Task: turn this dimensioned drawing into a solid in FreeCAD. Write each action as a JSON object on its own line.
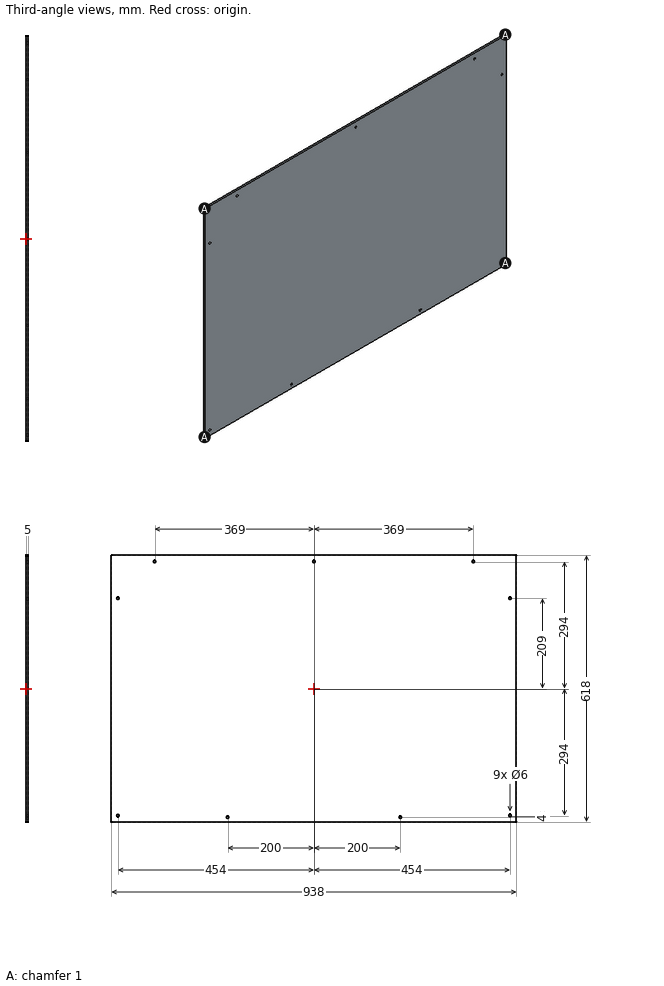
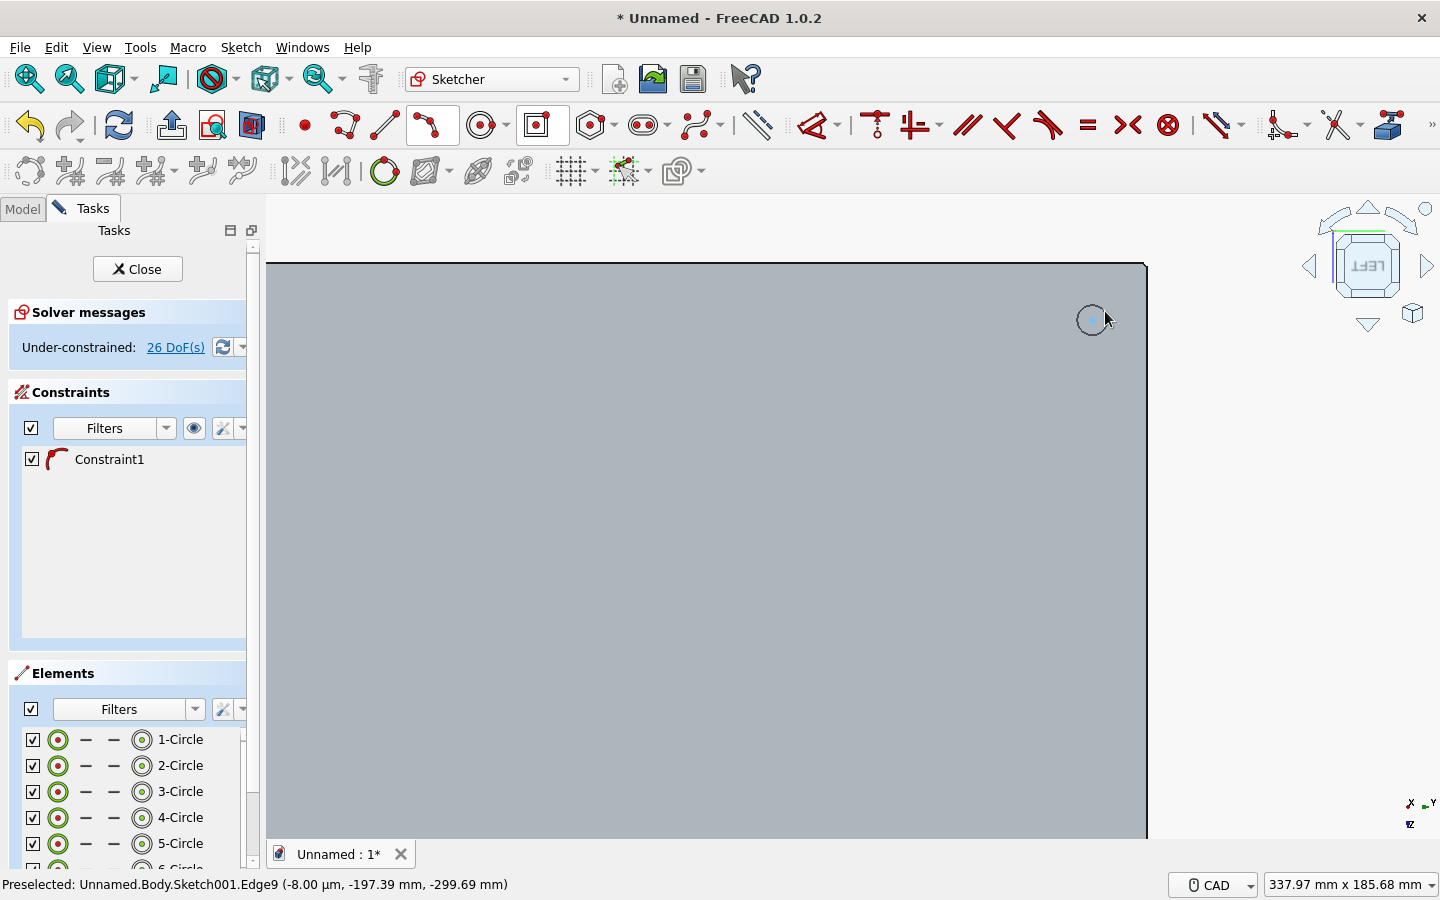
{"action": "left_click", "coordinate": [1103, 310]}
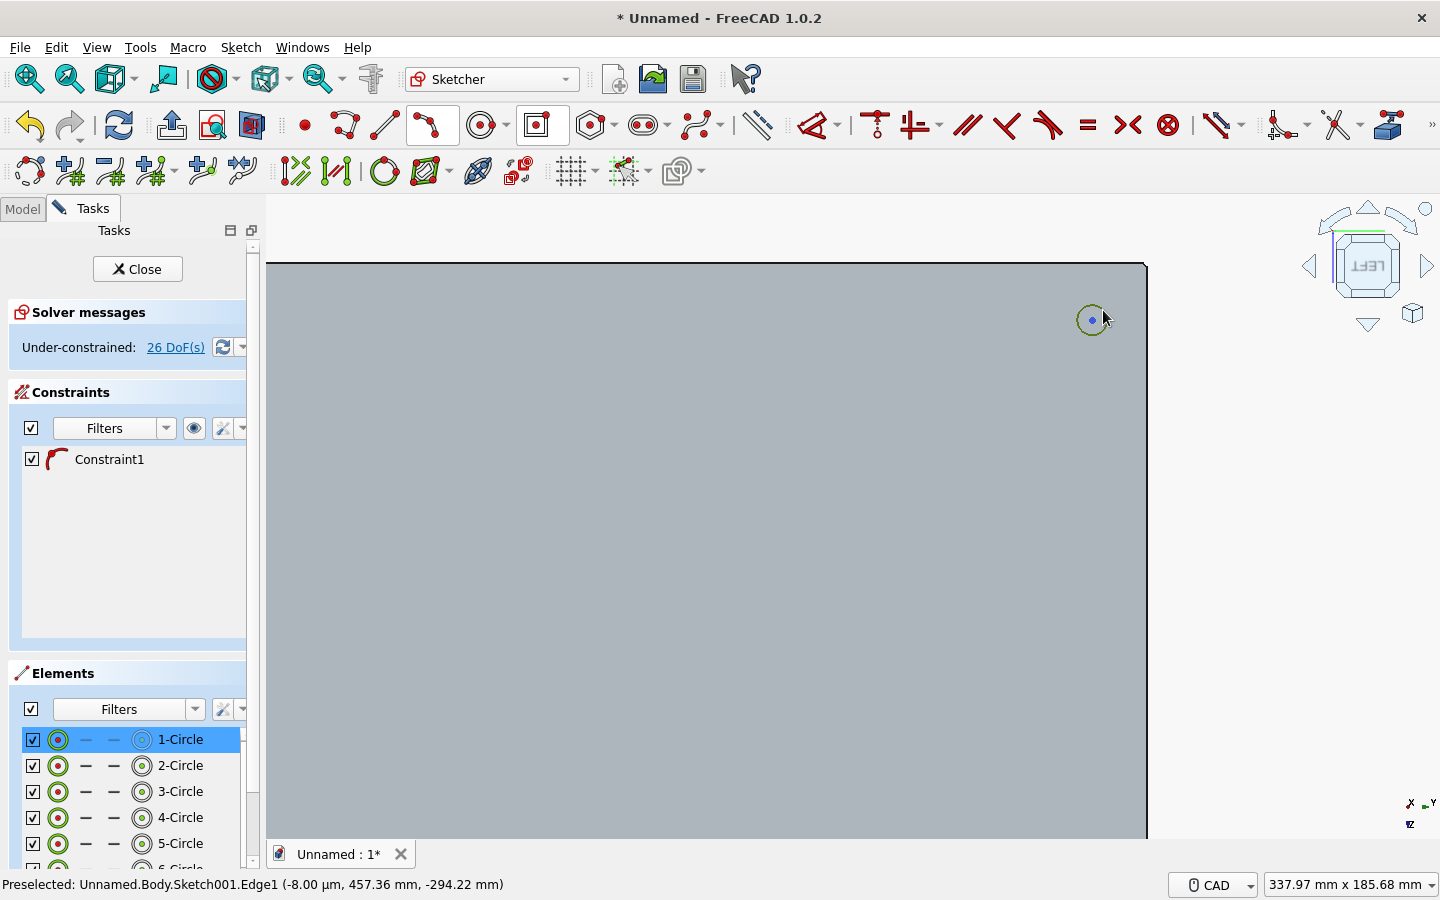
{"action": "scroll", "coordinate": [1105, 311], "scroll_direction": "down", "scroll_amount": 8}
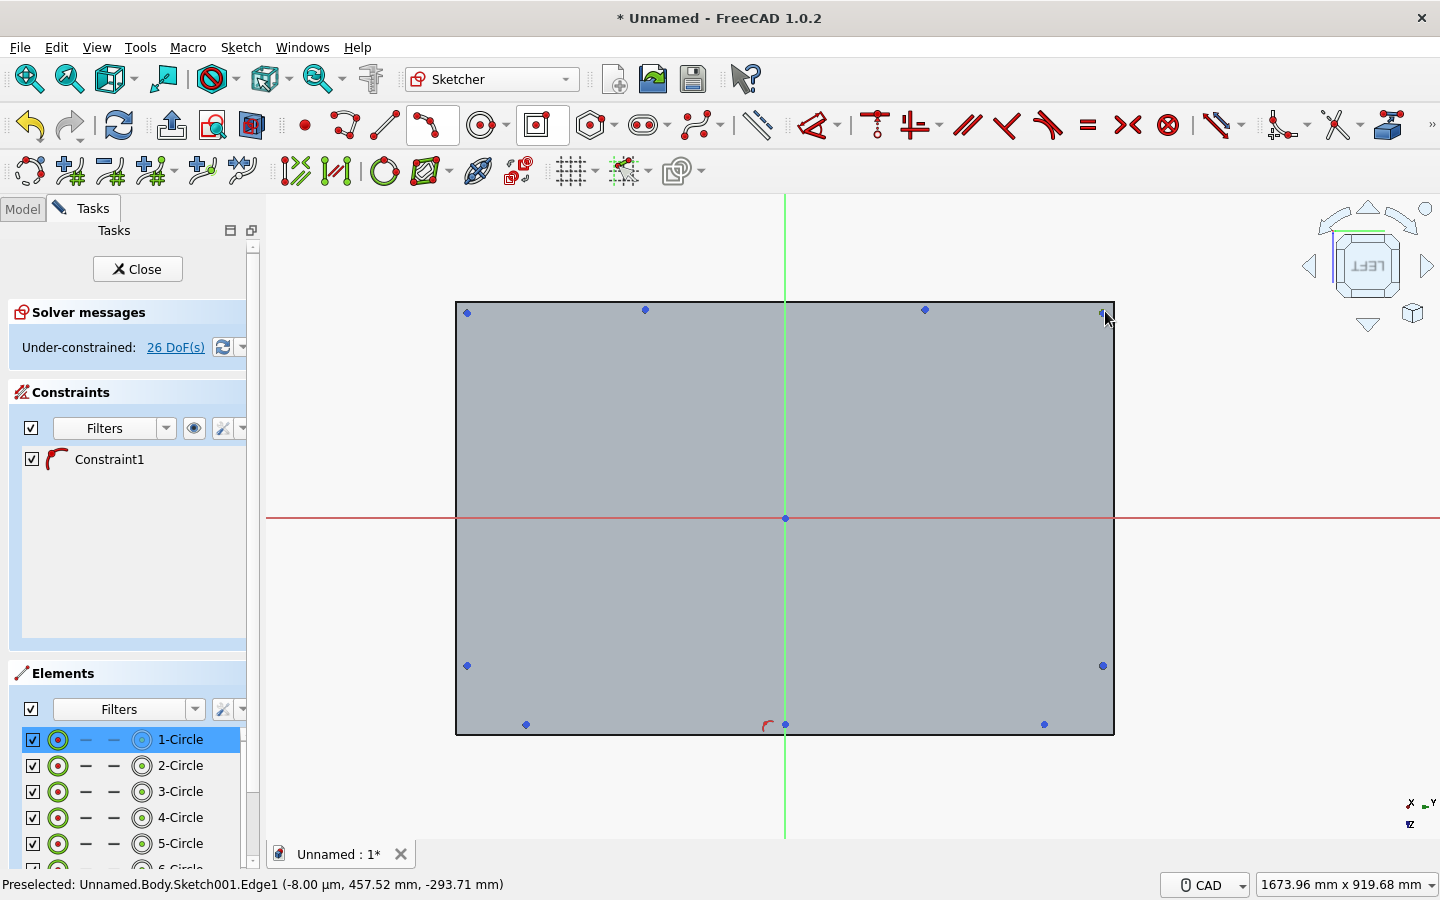
{"action": "scroll", "coordinate": [469, 311], "scroll_direction": "up", "scroll_amount": 9}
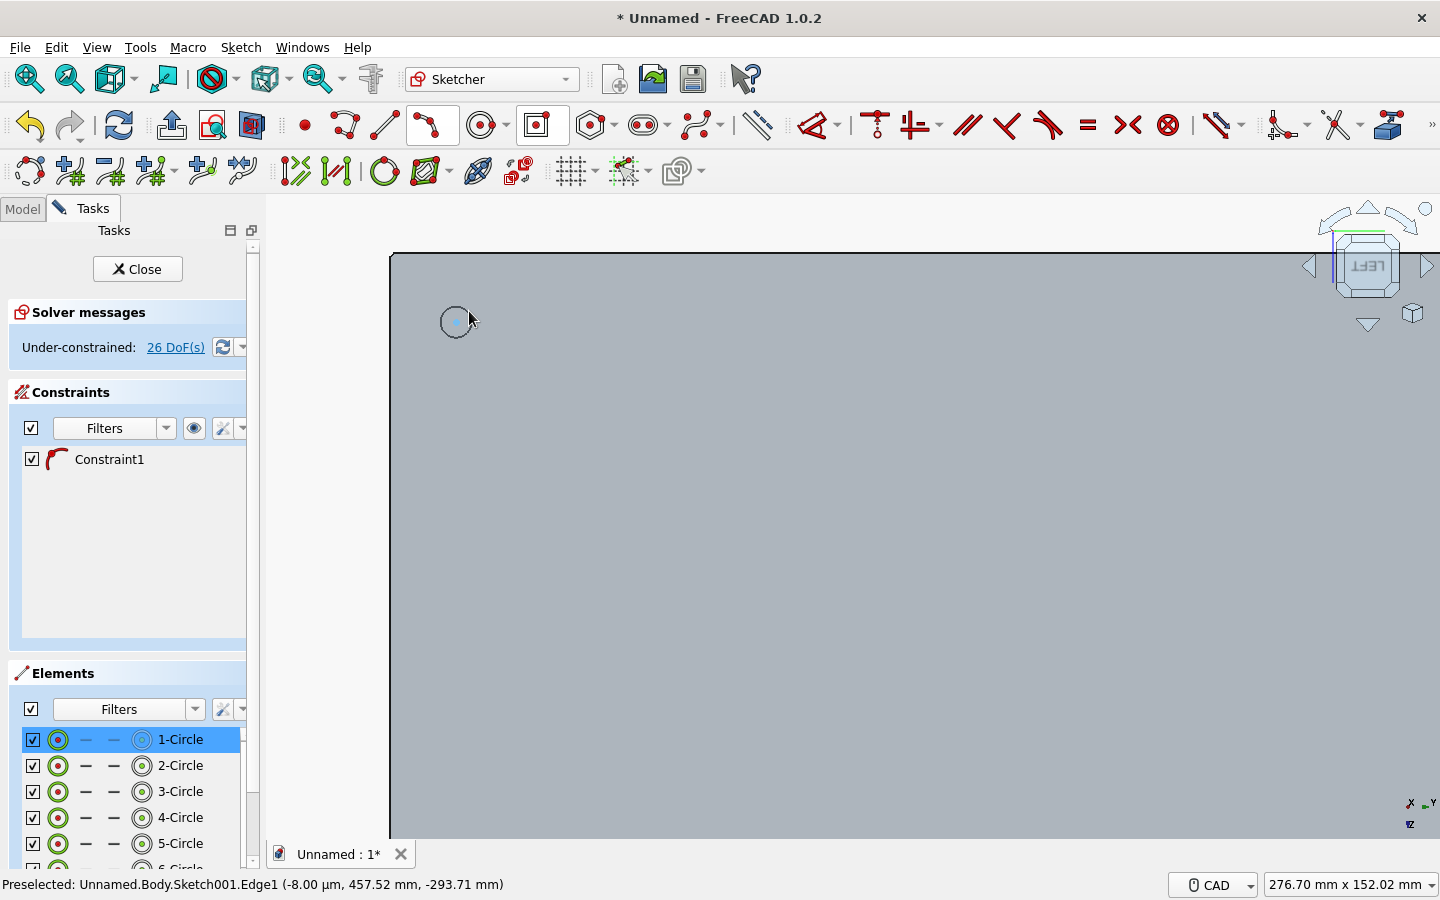
{"action": "left_click", "coordinate": [467, 311]}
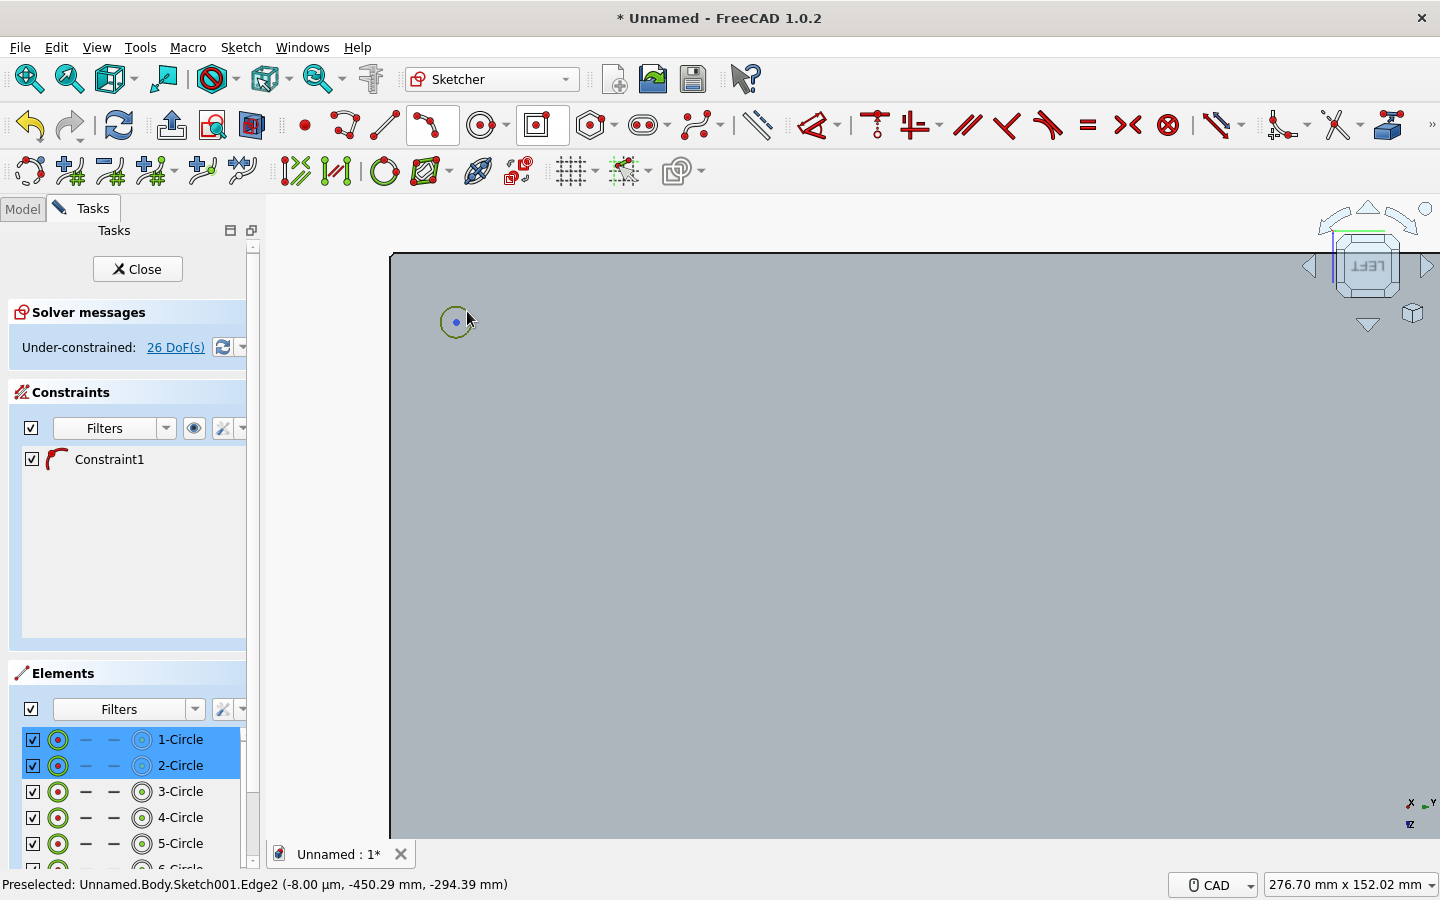
{"action": "scroll", "coordinate": [469, 311], "scroll_direction": "down", "scroll_amount": 9}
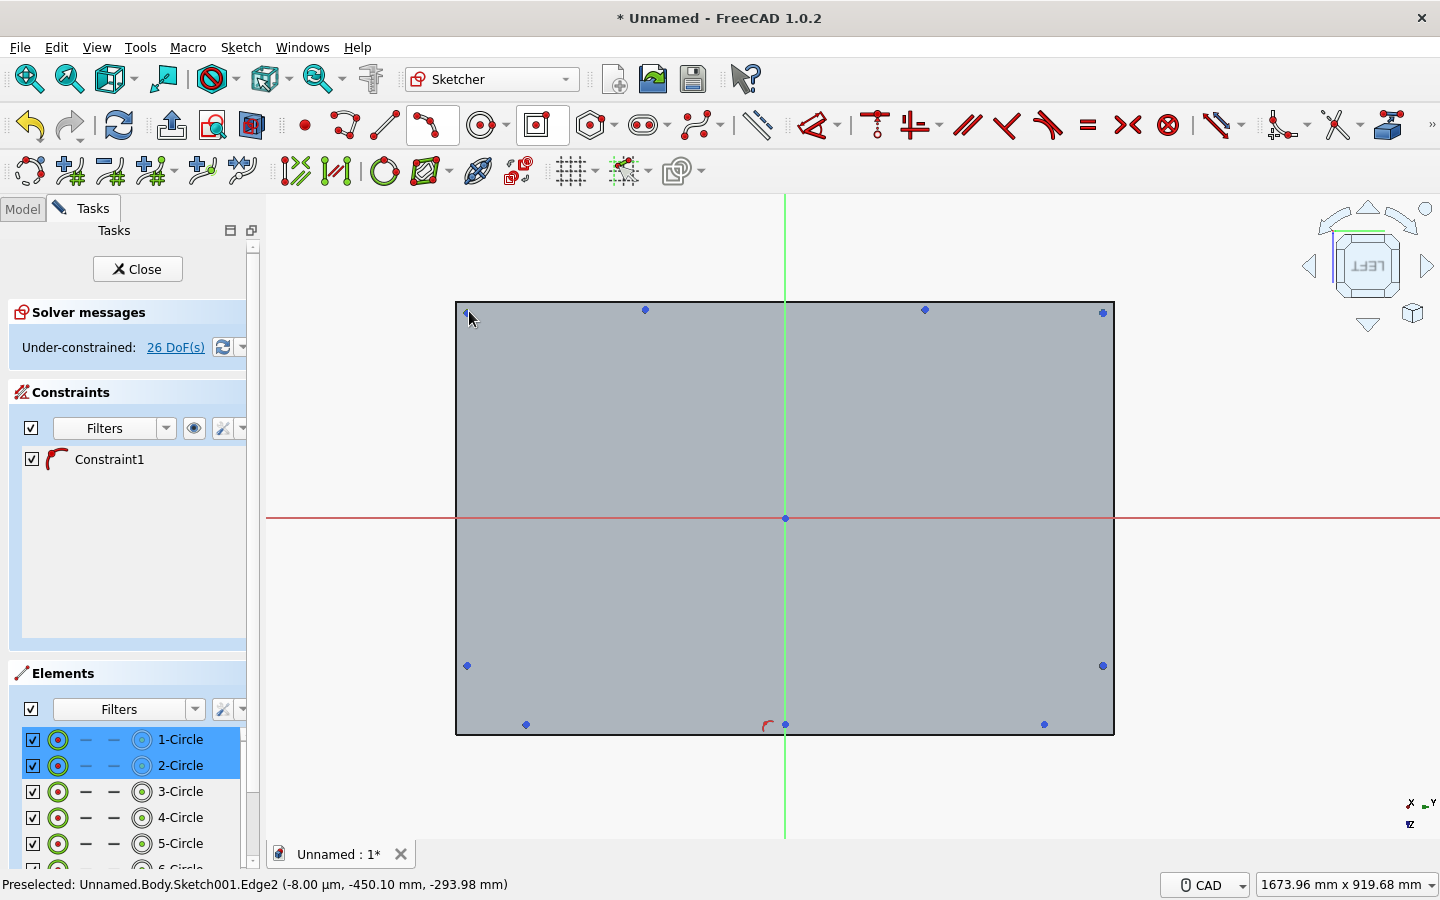
{"action": "scroll", "coordinate": [1105, 664], "scroll_direction": "up", "scroll_amount": 8}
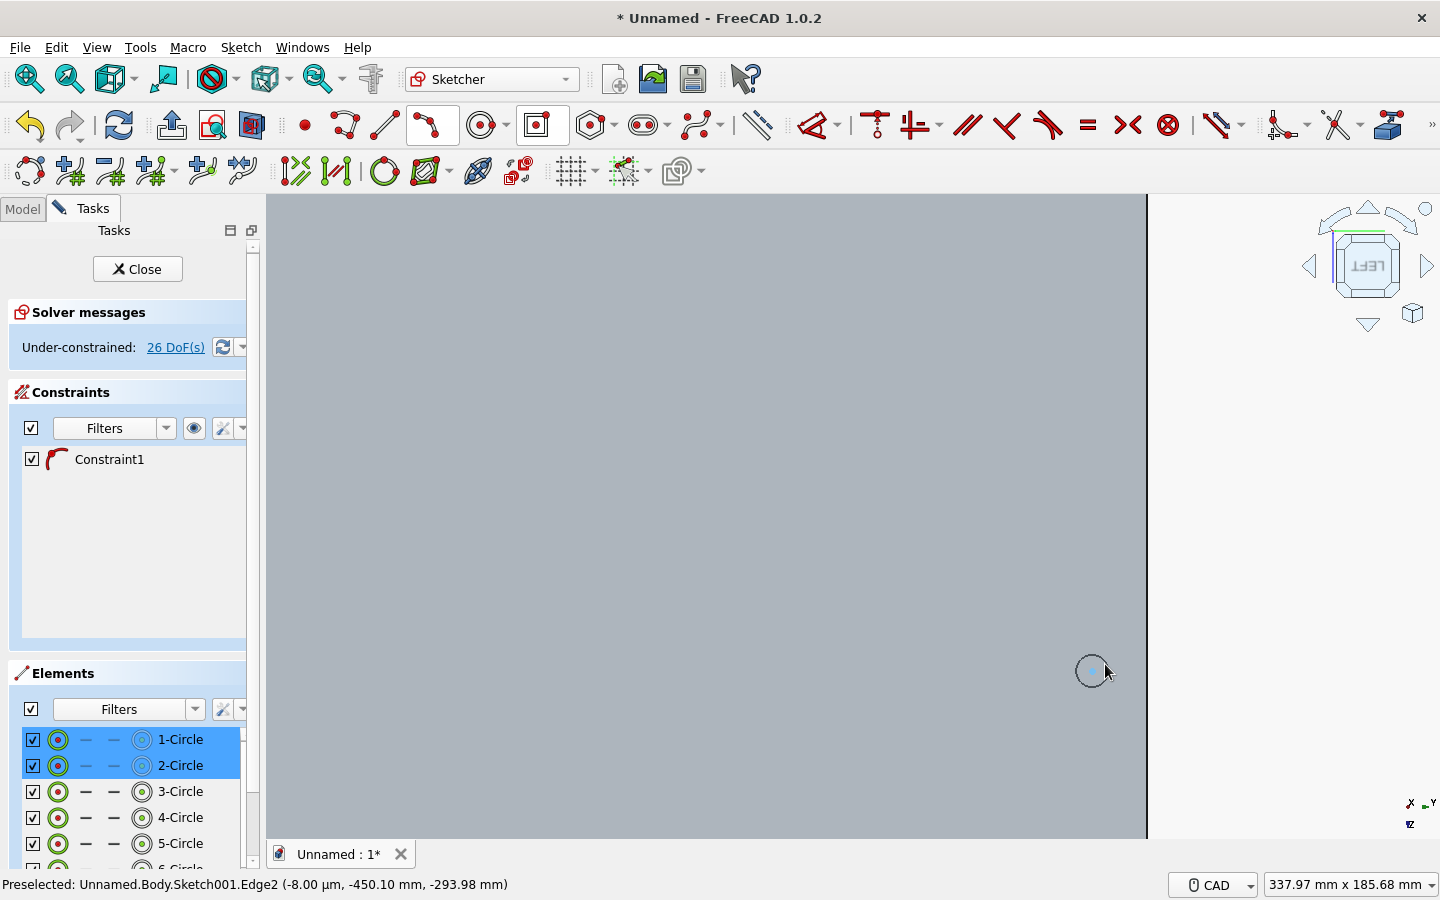
{"action": "left_click", "coordinate": [1104, 660]}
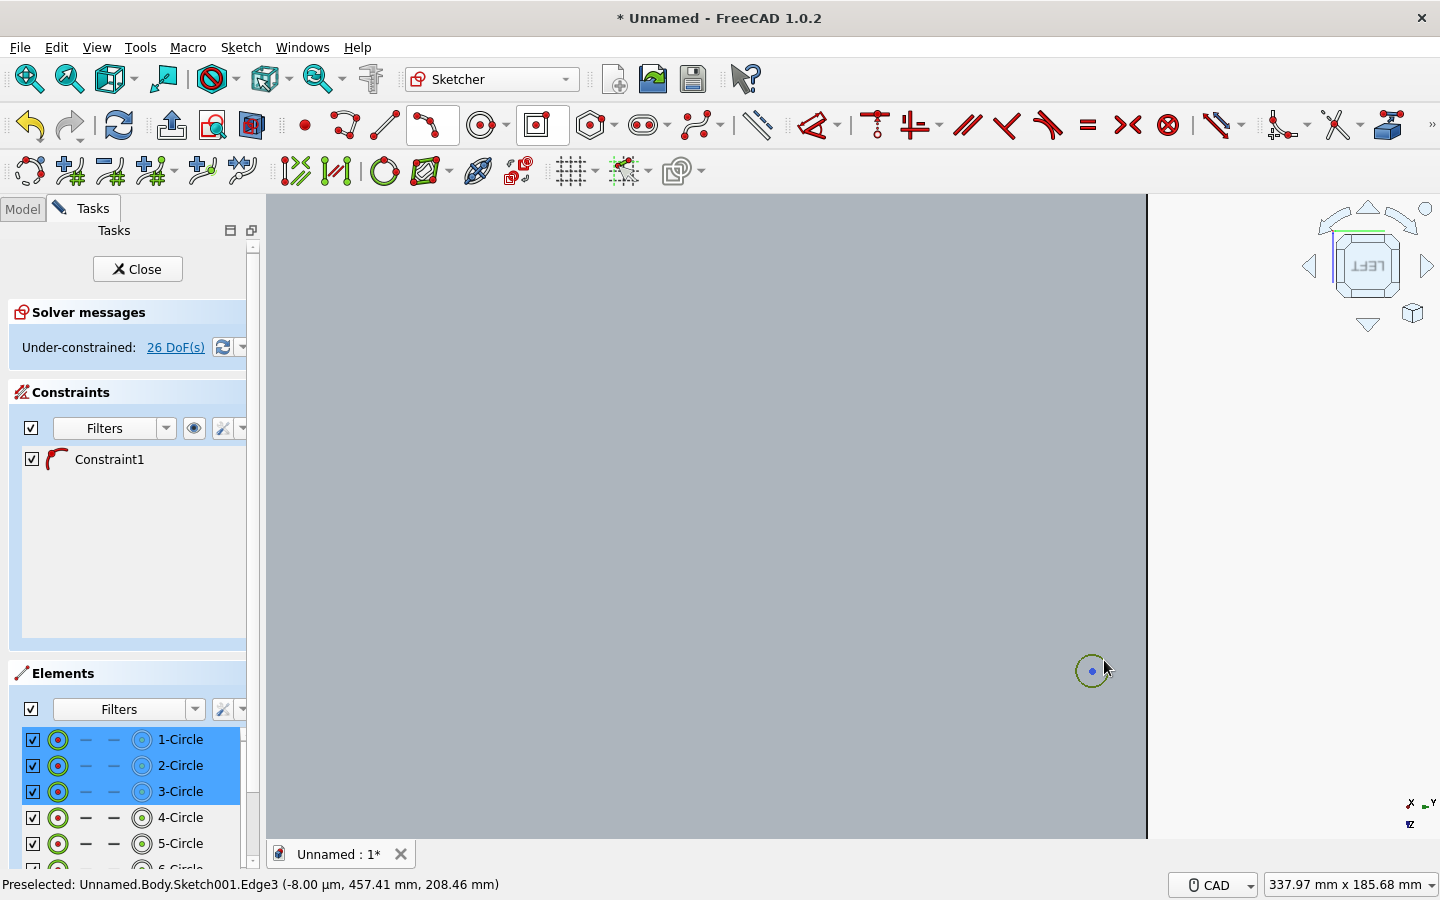
{"action": "scroll", "coordinate": [1105, 664], "scroll_direction": "down", "scroll_amount": 8}